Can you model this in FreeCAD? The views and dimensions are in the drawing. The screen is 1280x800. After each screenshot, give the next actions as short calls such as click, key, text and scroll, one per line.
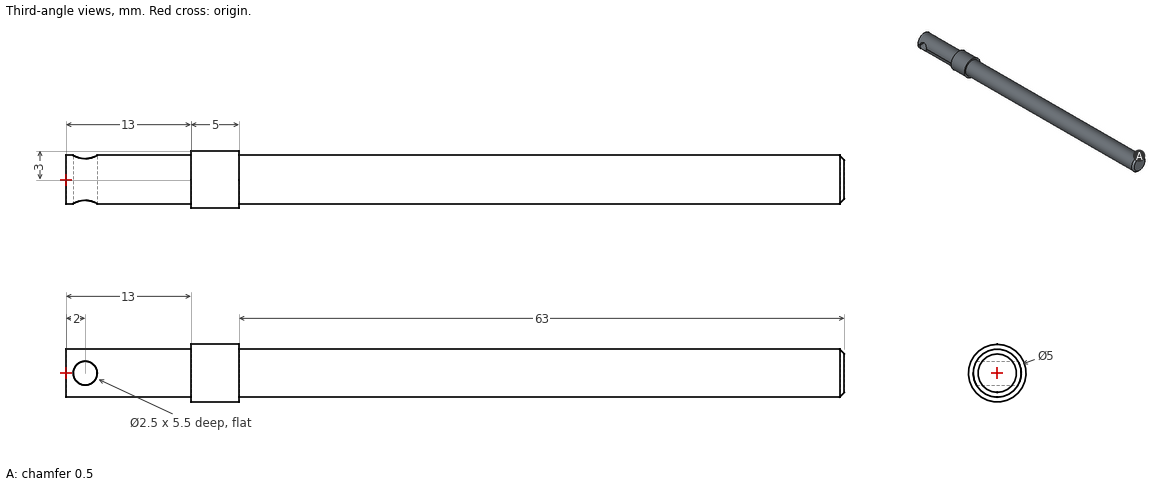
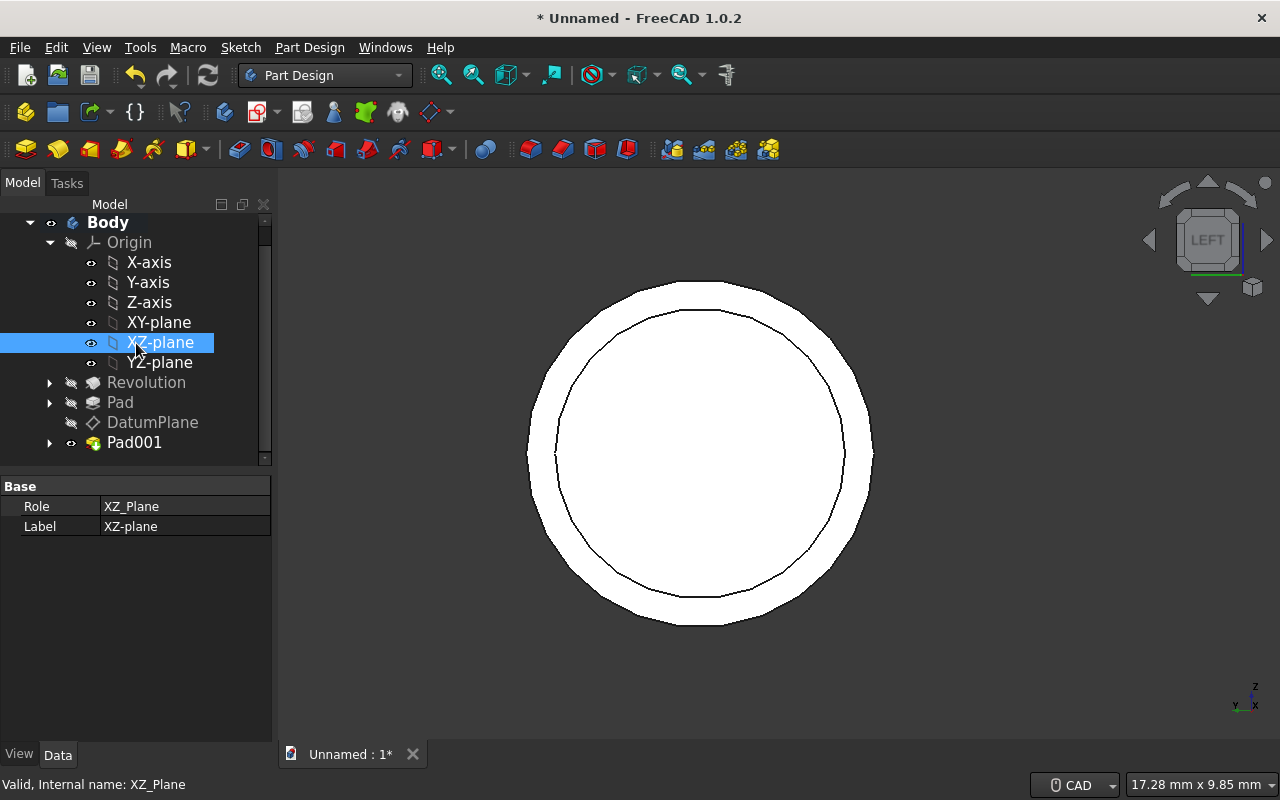
click(430, 112)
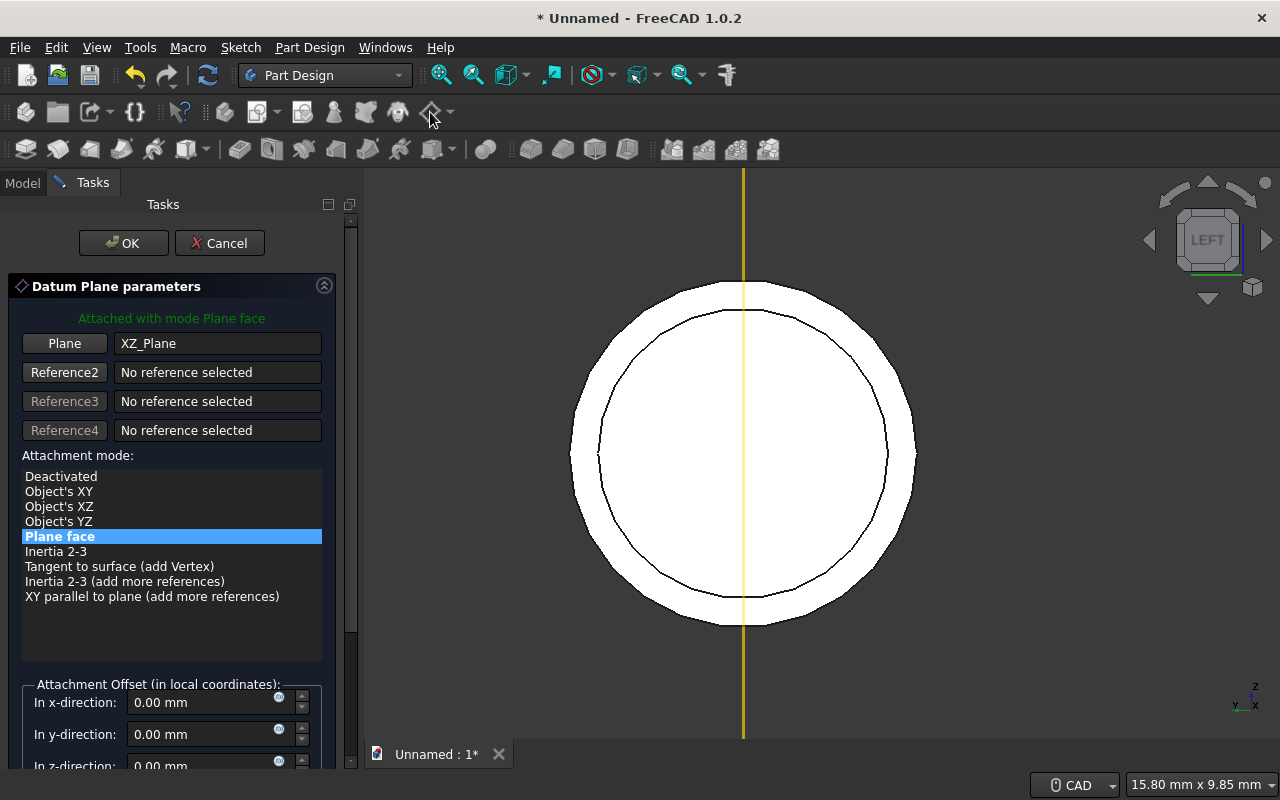
scroll(351, 491, down, 2)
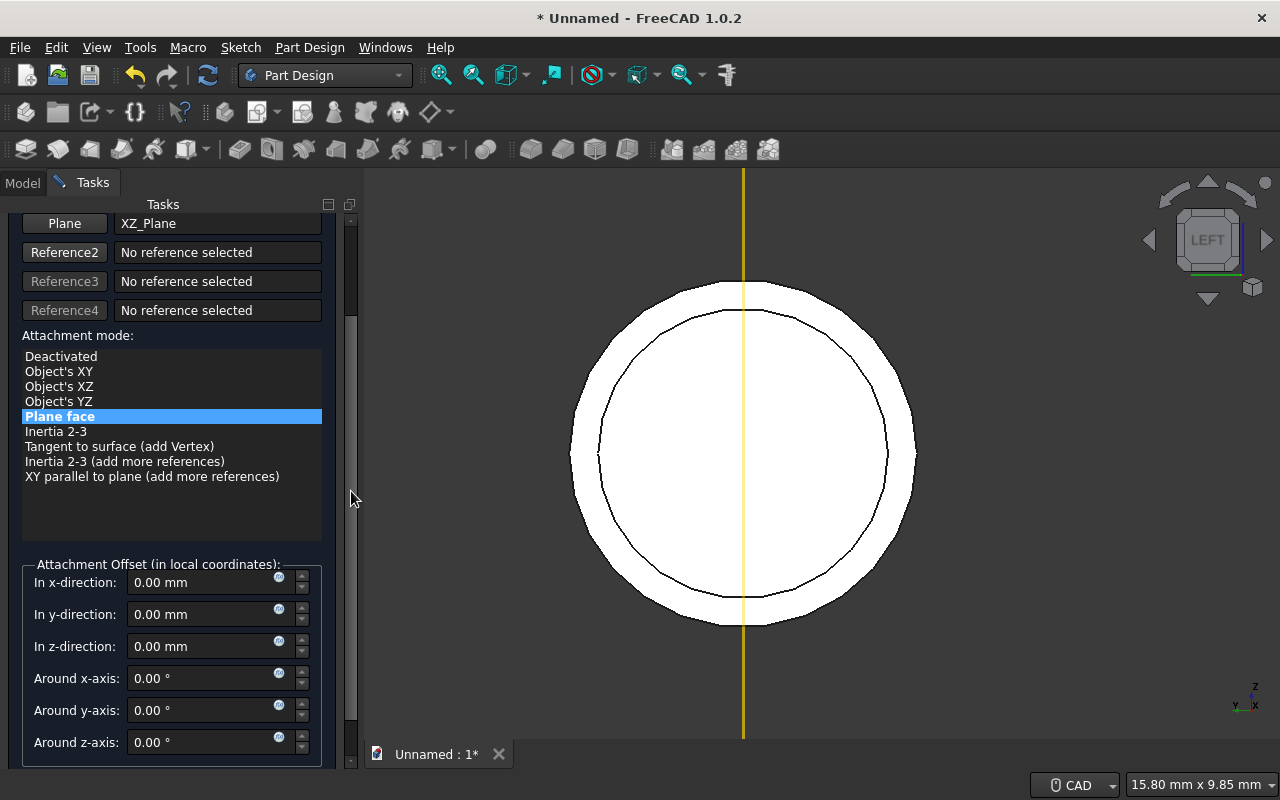
triple_click(210, 646)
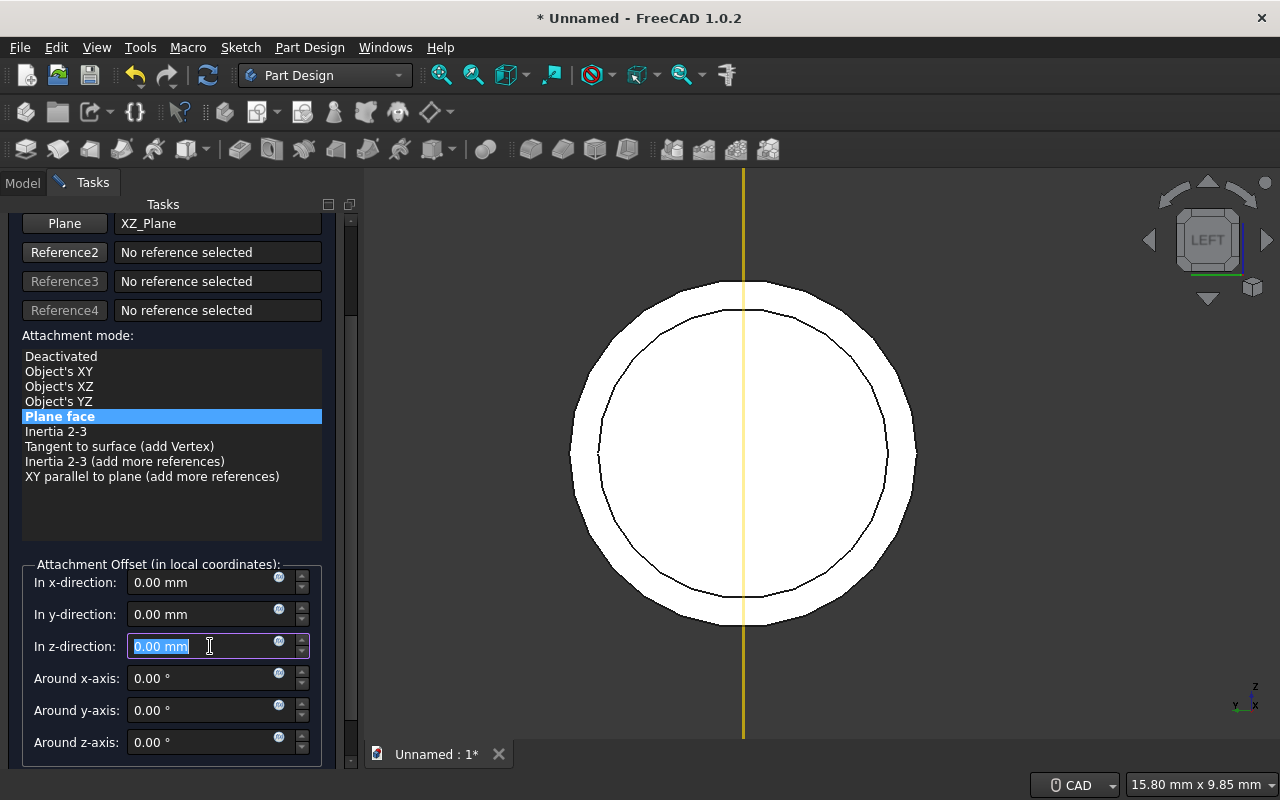
text(2.5)
key(Tab)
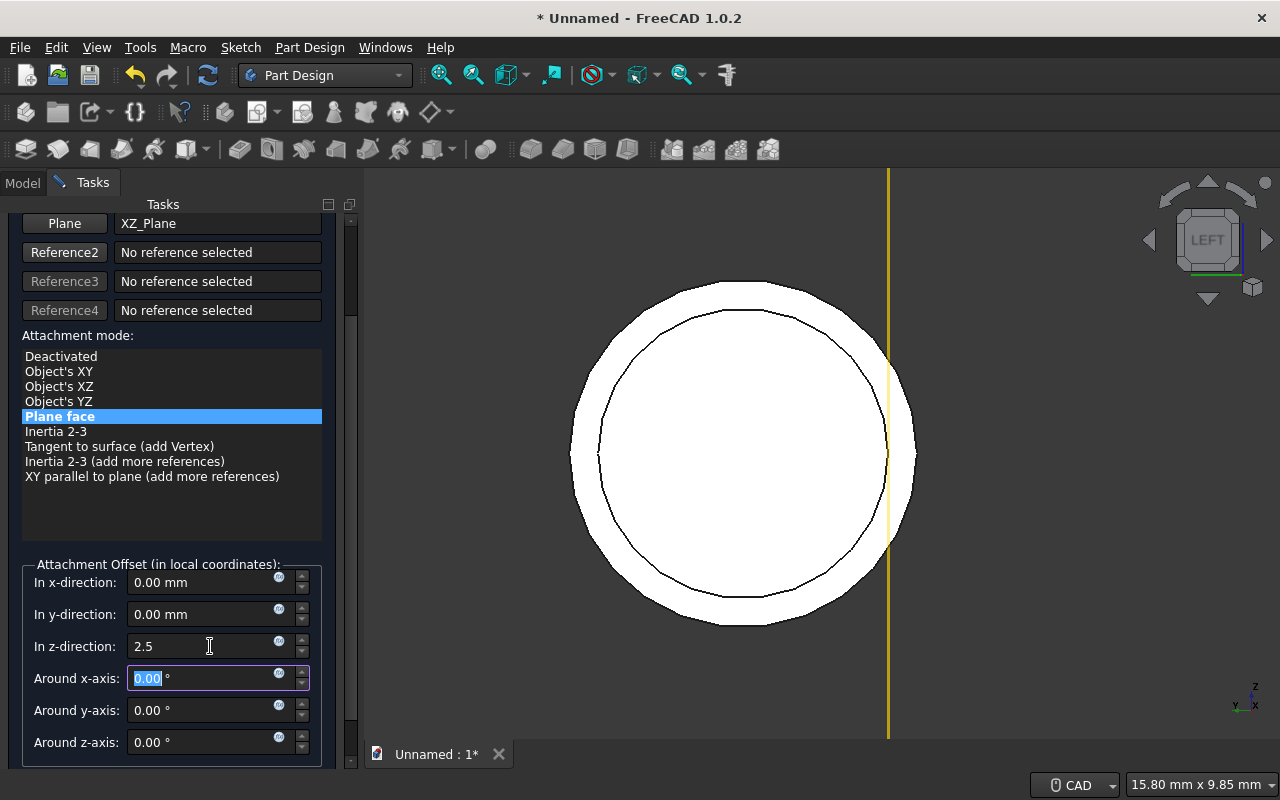
scroll(351, 491, up, 3)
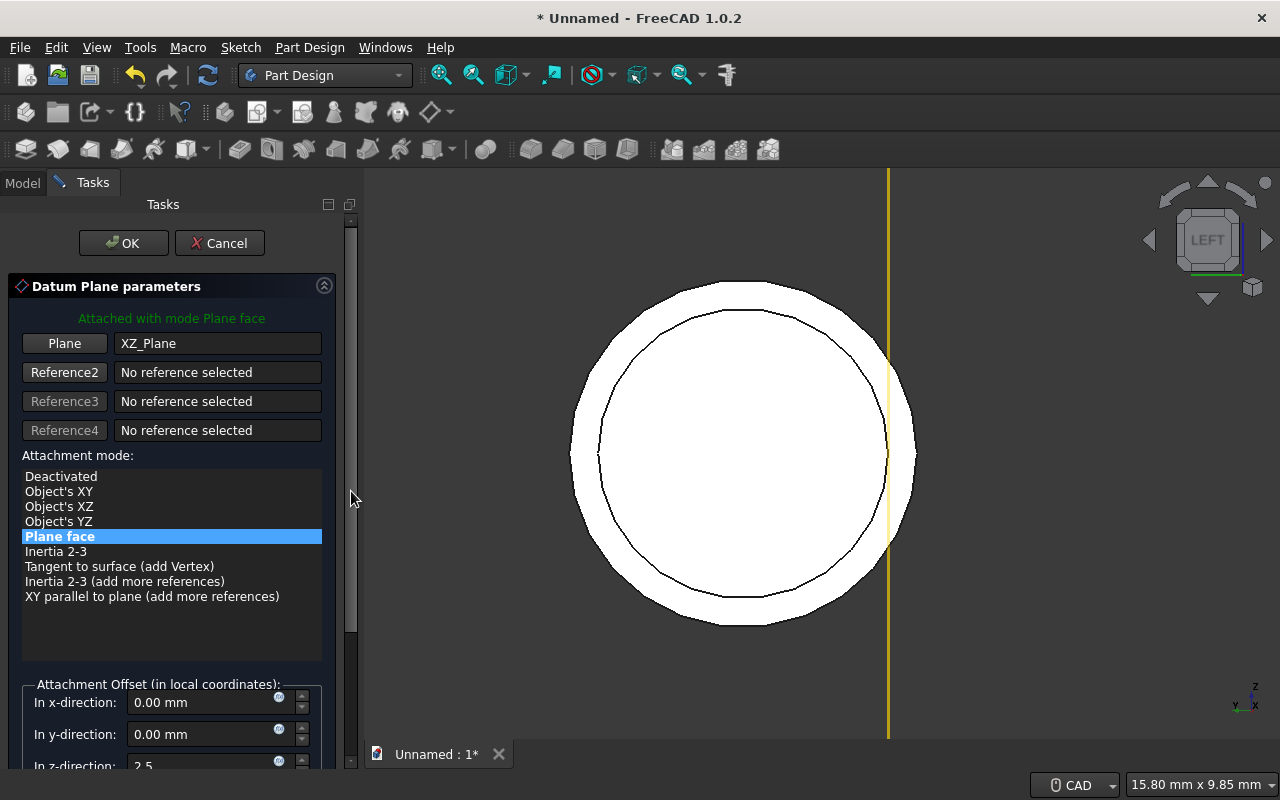
click(124, 243)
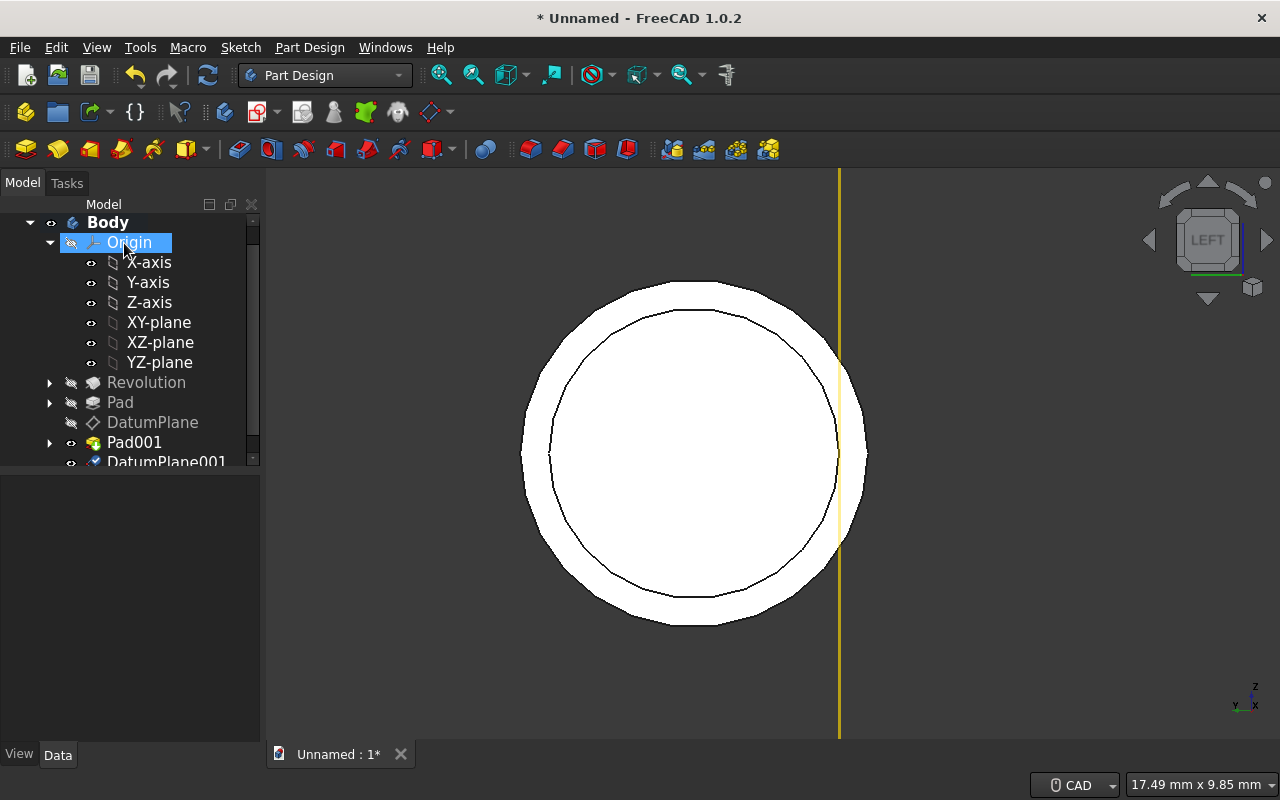
click(116, 463)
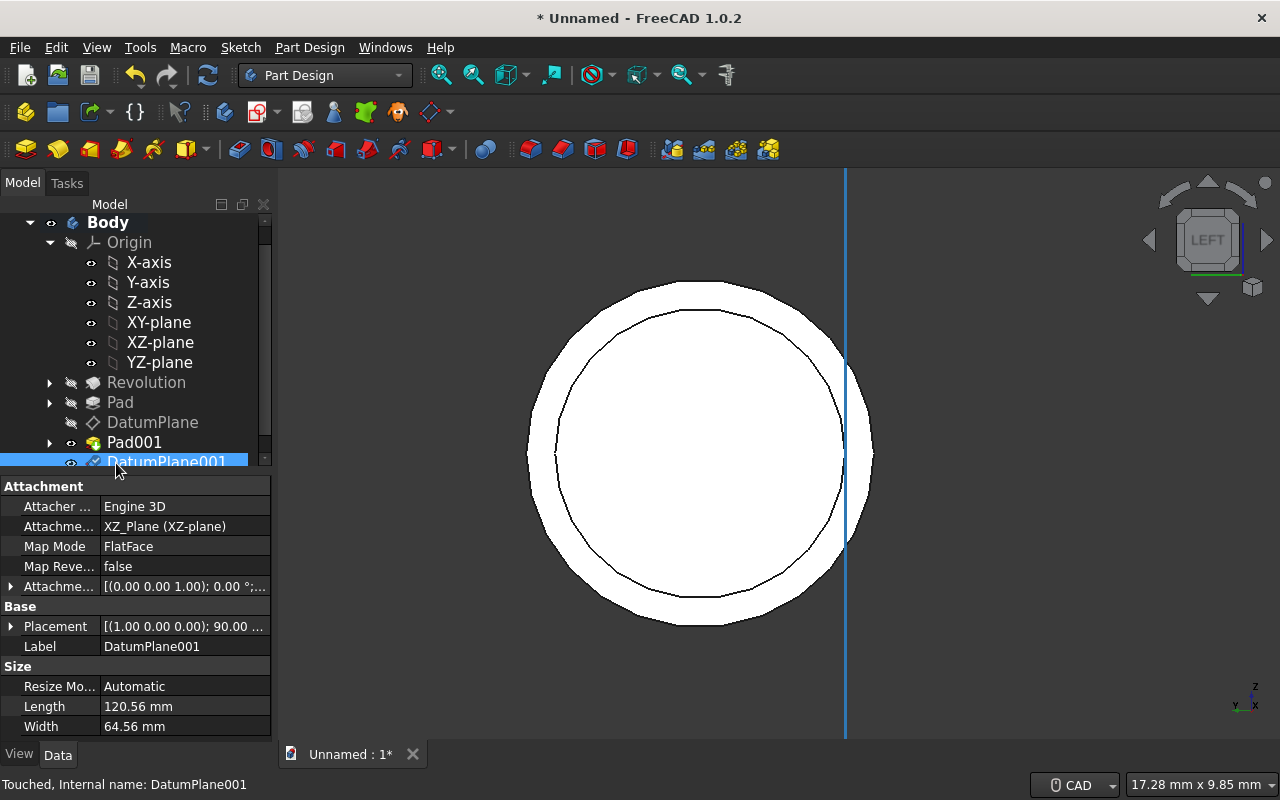
click(258, 112)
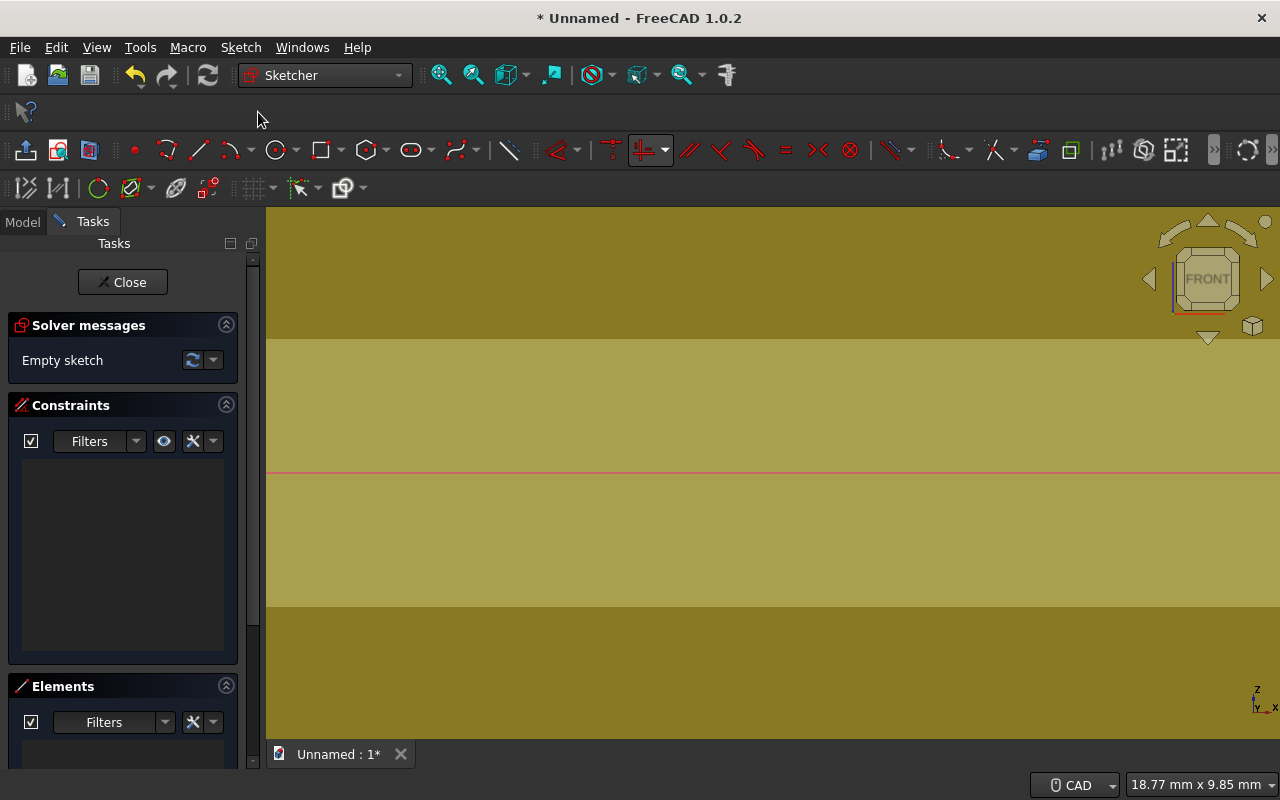
click(90, 150)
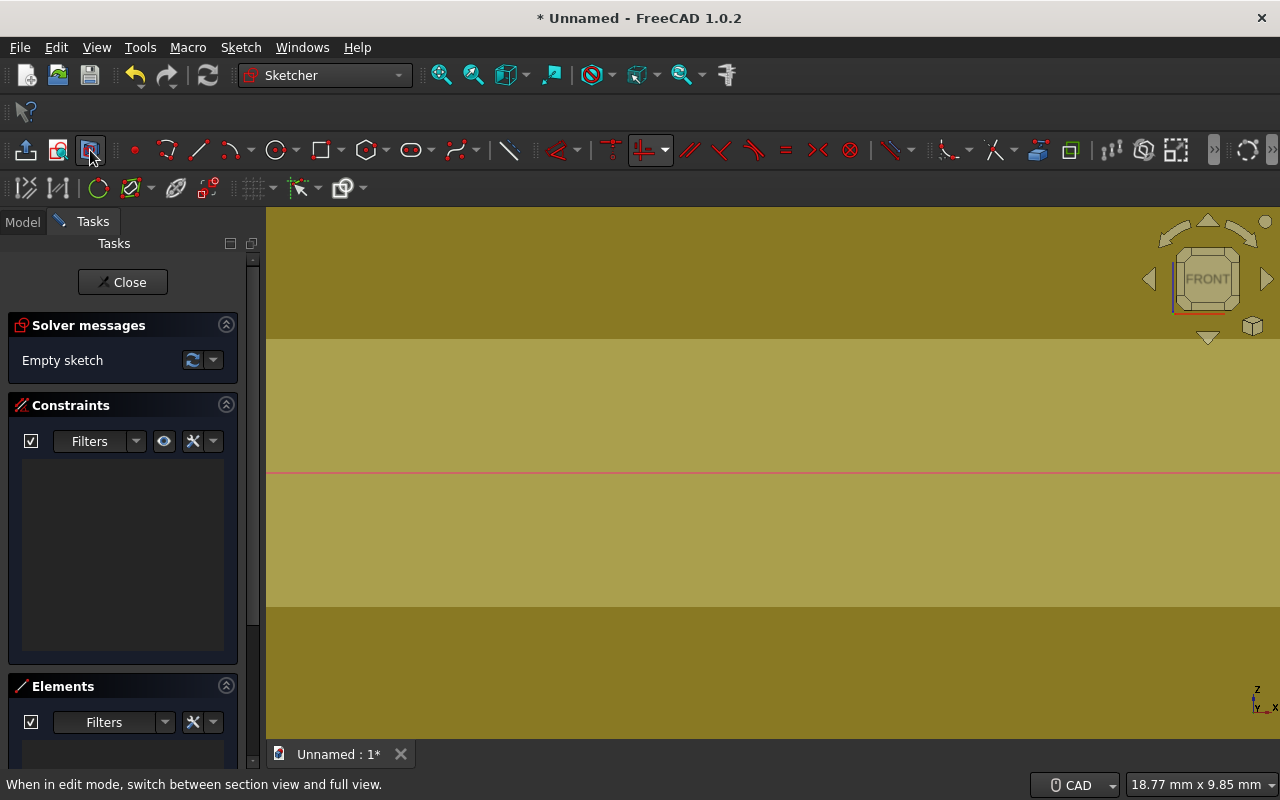
scroll(704, 473, down, 5)